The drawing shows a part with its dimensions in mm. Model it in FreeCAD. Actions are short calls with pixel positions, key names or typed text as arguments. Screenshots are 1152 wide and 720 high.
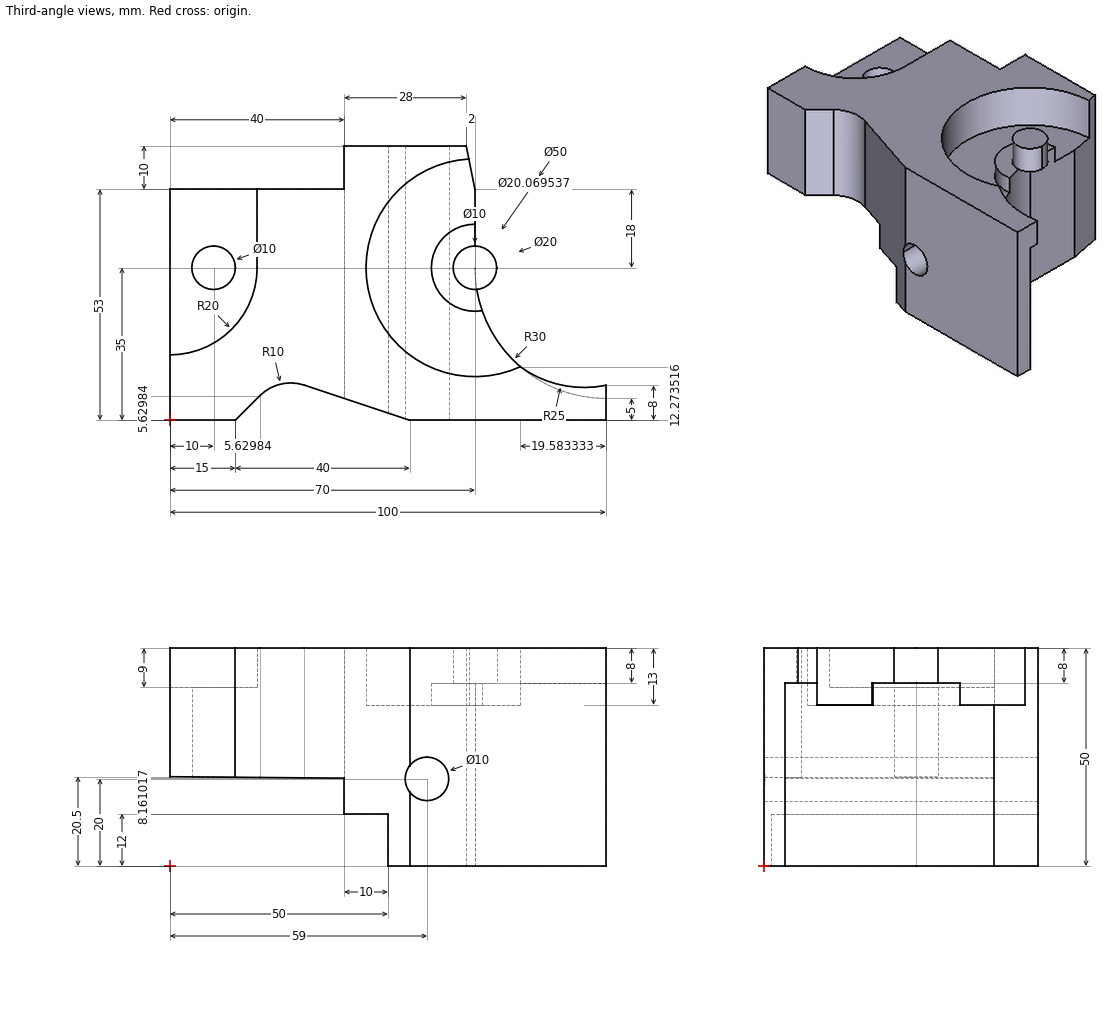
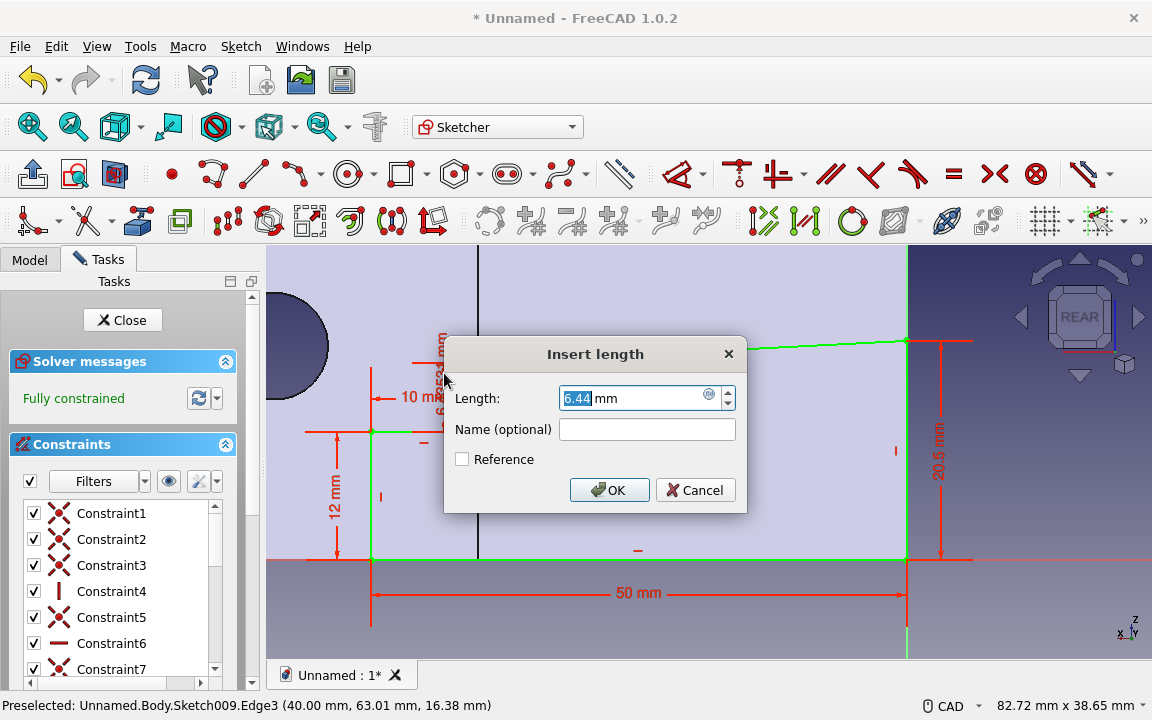
text(8.161017)
key(Return)
key(Escape)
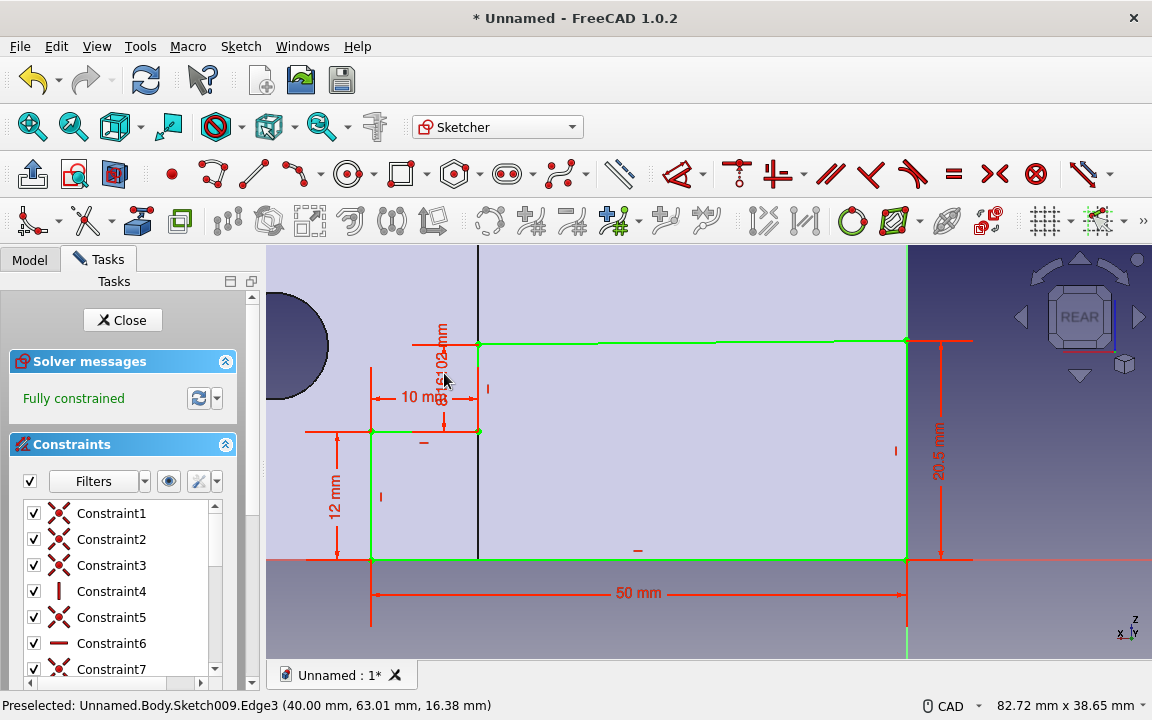
click(123, 320)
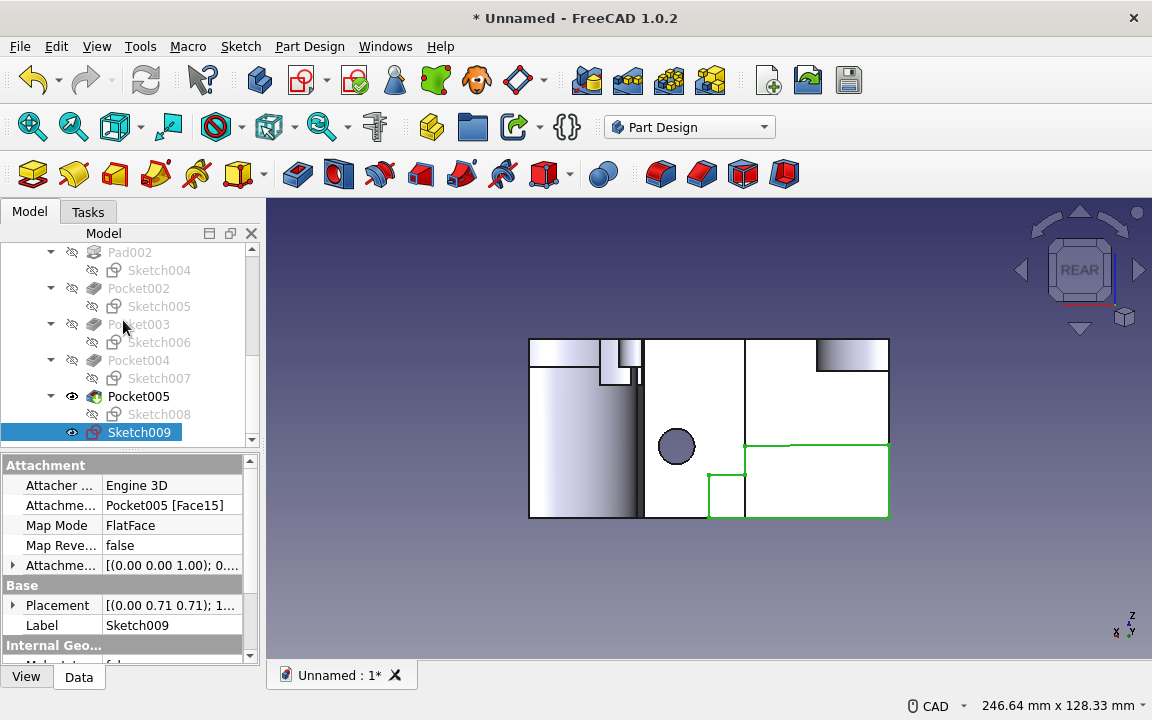
click(298, 174)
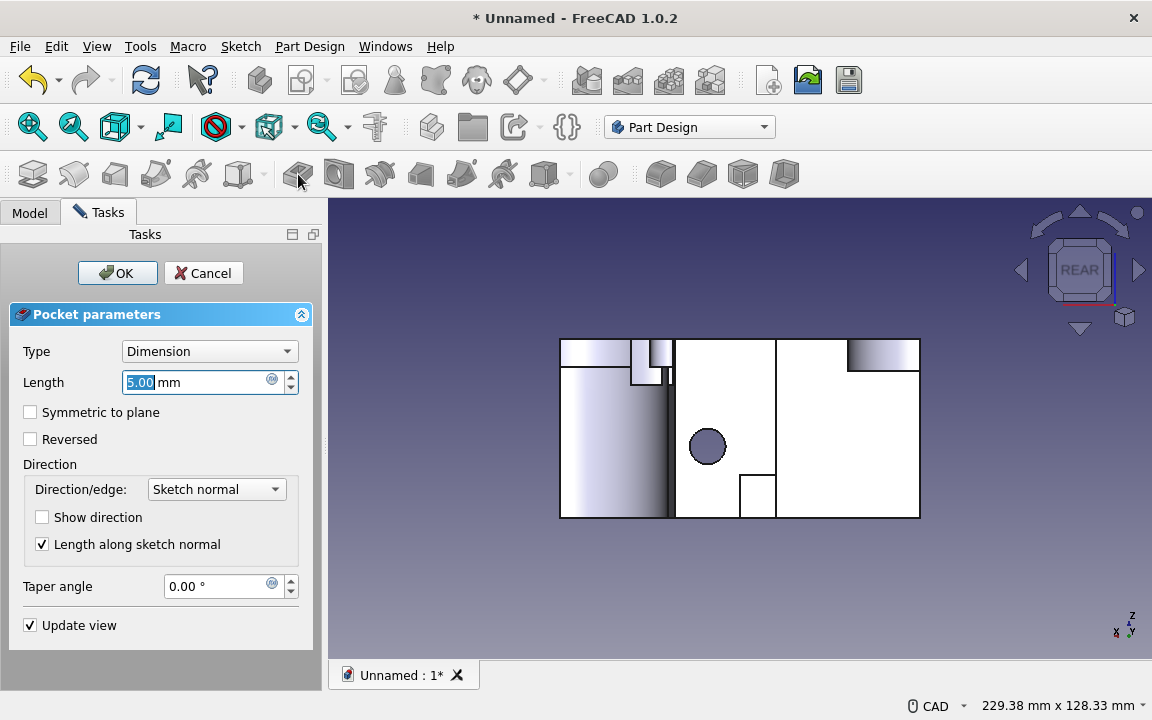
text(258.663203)
key(Tab)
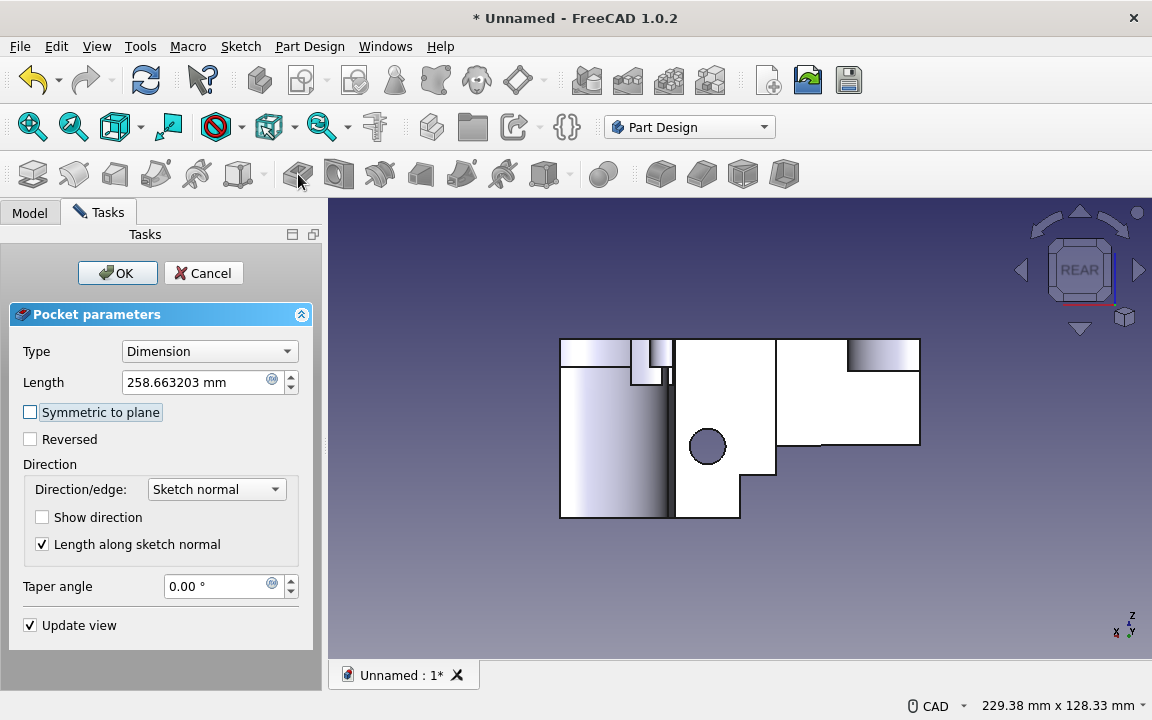
click(31, 412)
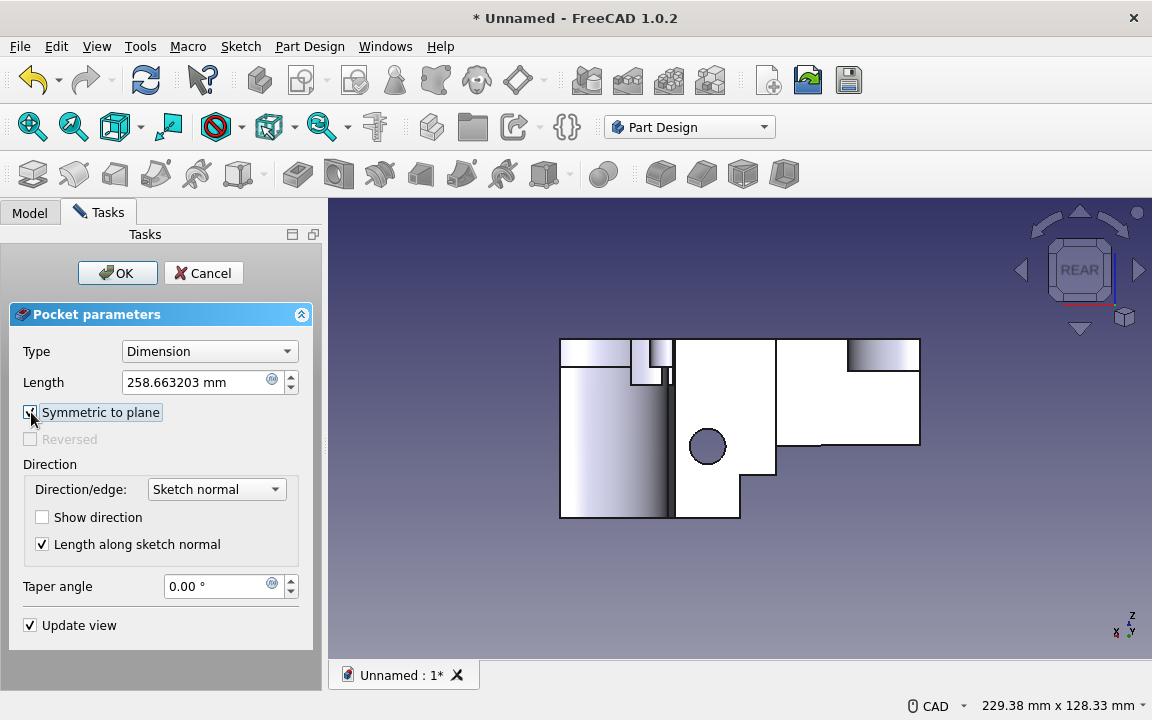
click(118, 273)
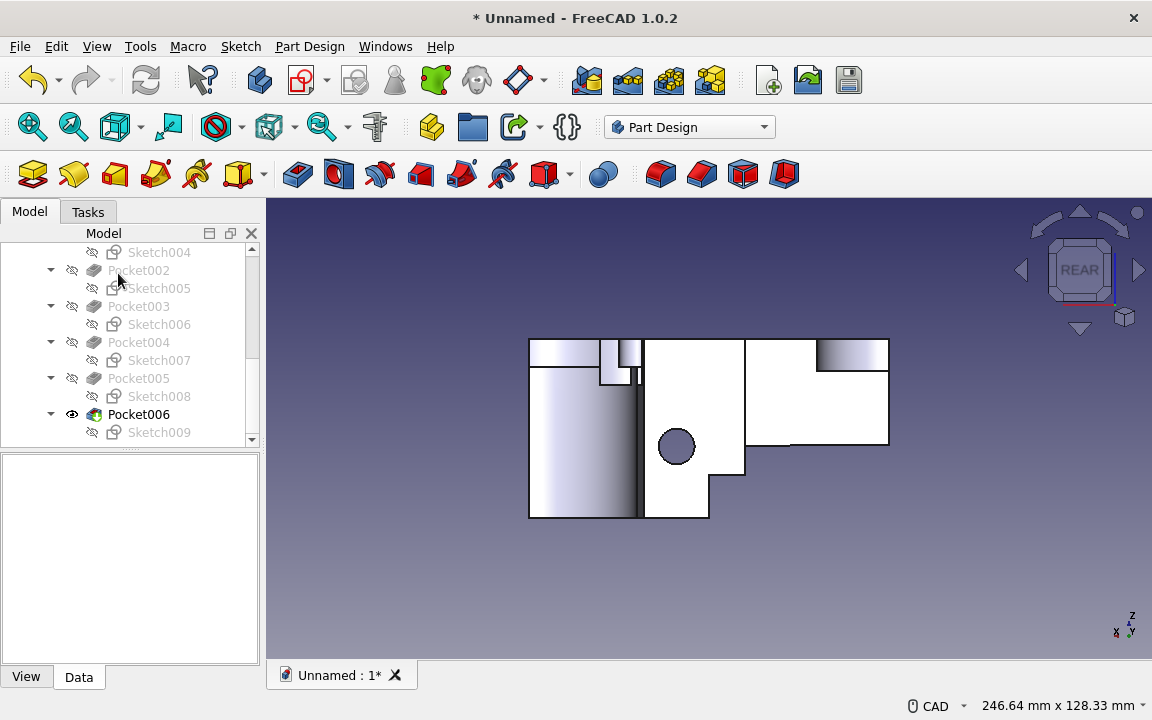
key(0)